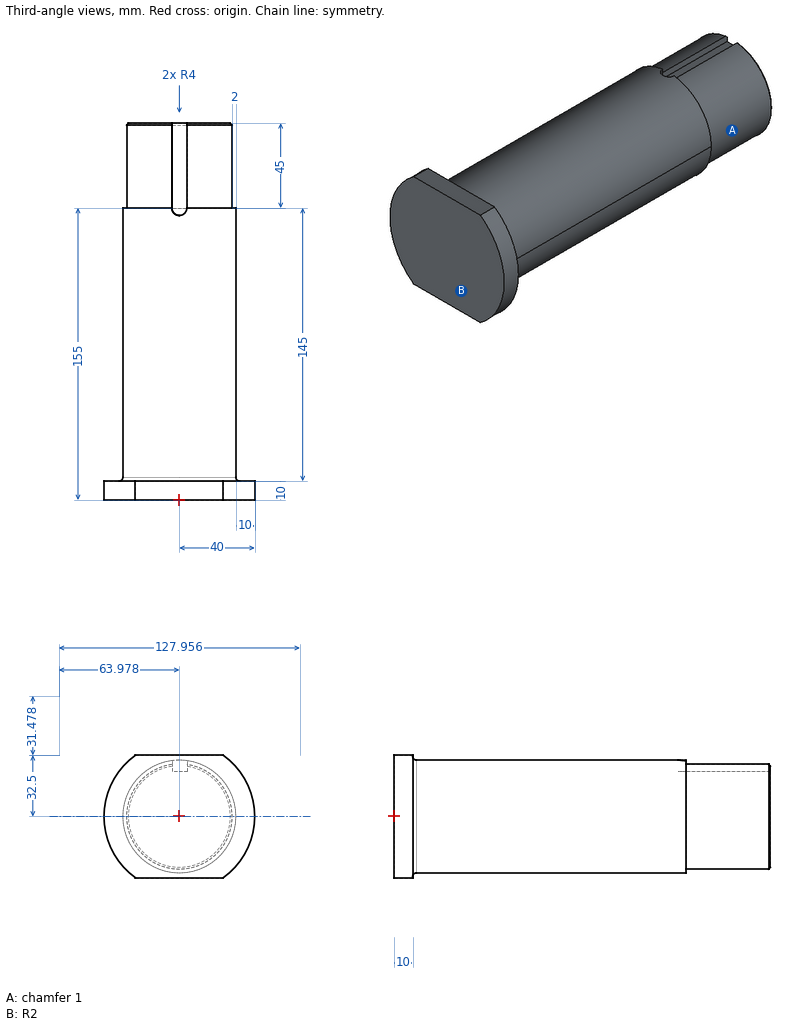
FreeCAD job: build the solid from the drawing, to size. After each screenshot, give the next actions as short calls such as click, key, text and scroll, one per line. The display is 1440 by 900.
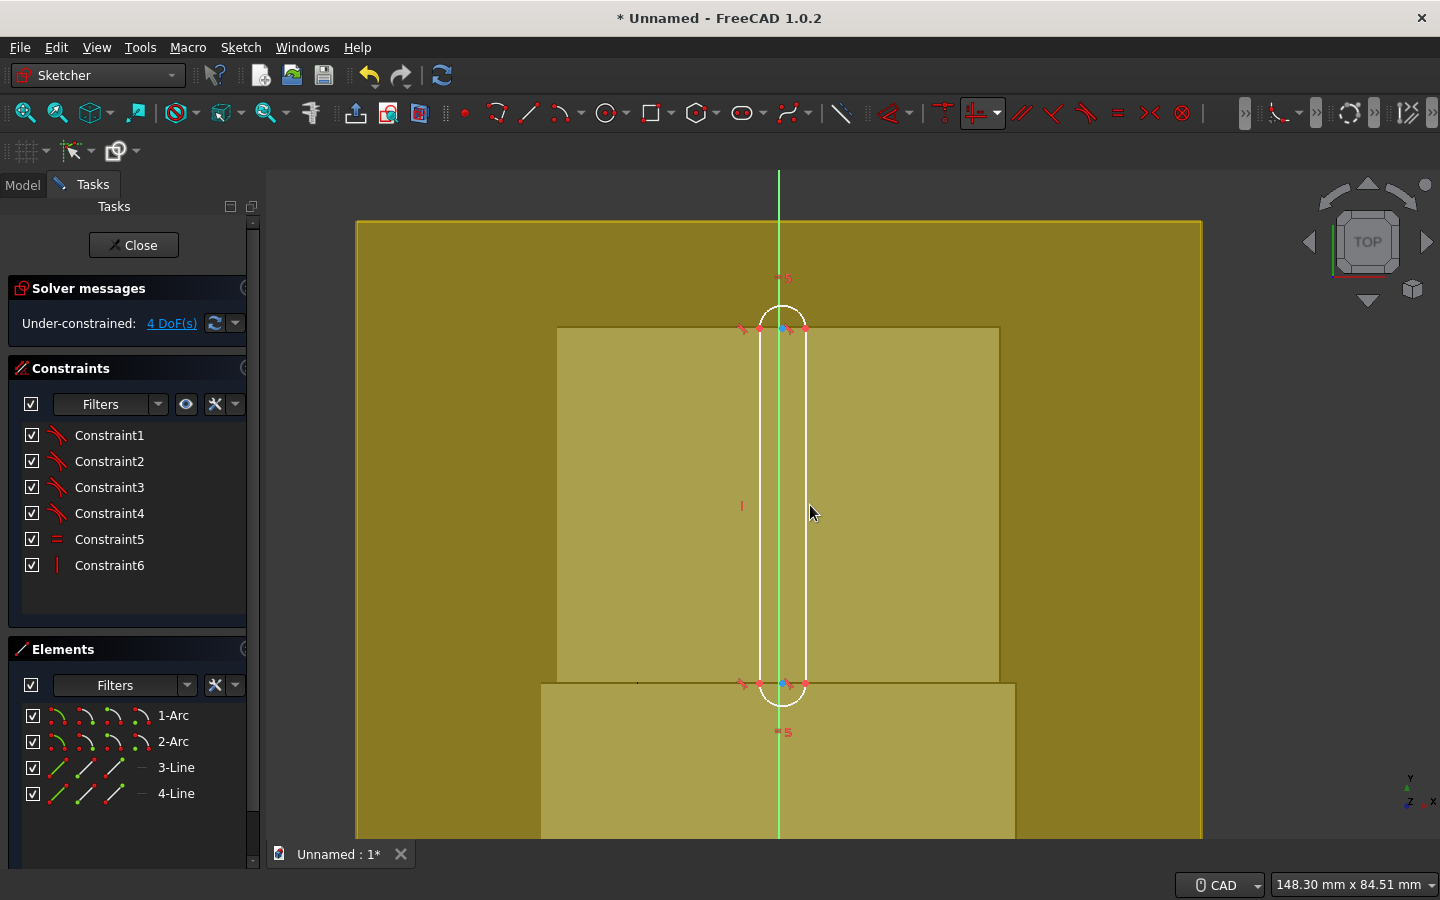
click(783, 683)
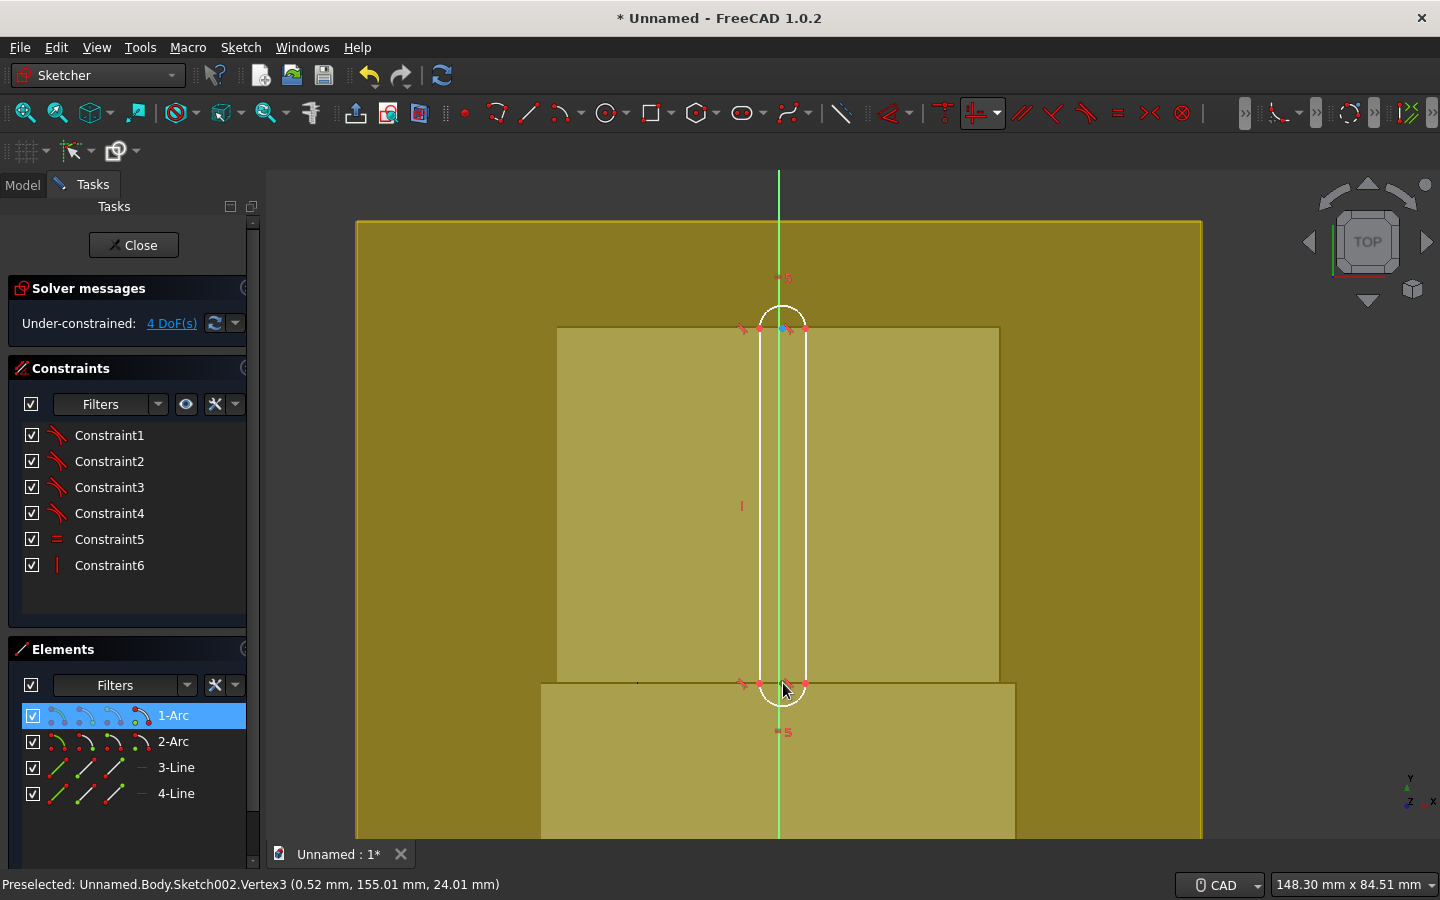
click(779, 767)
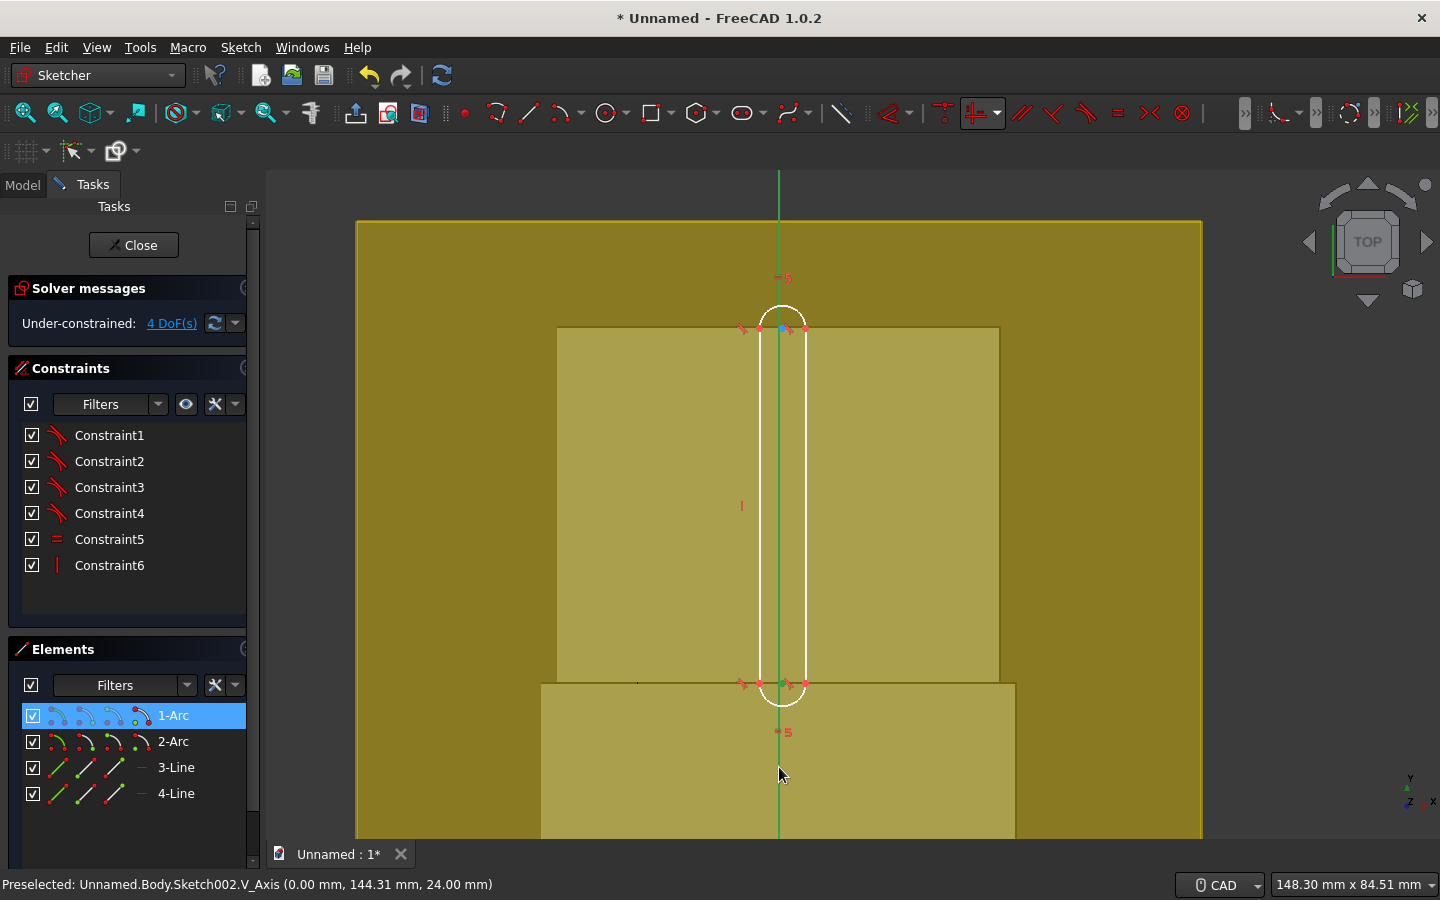
click(944, 114)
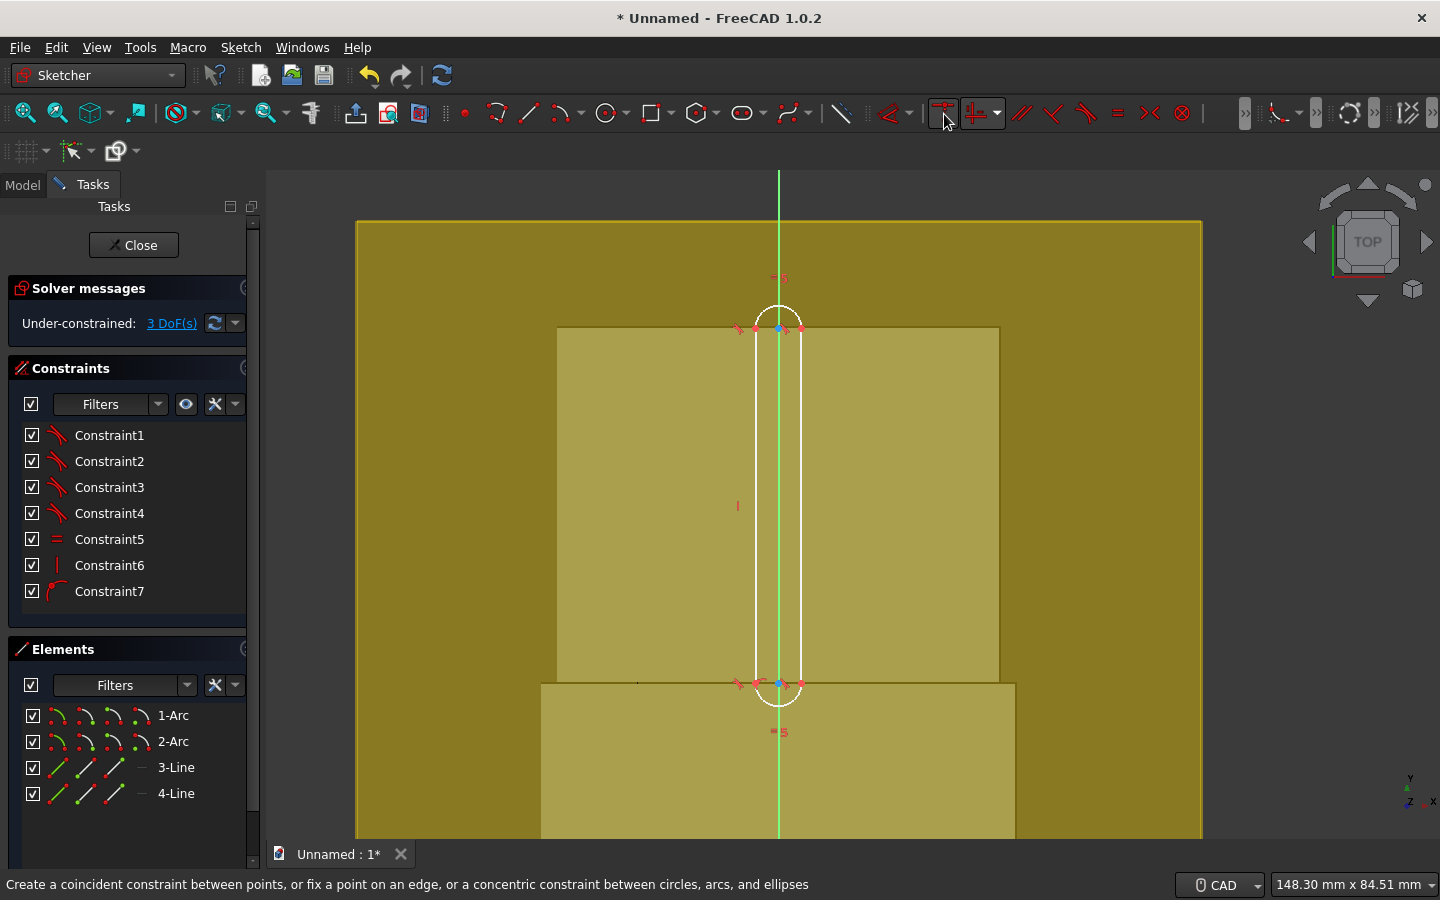
click(888, 114)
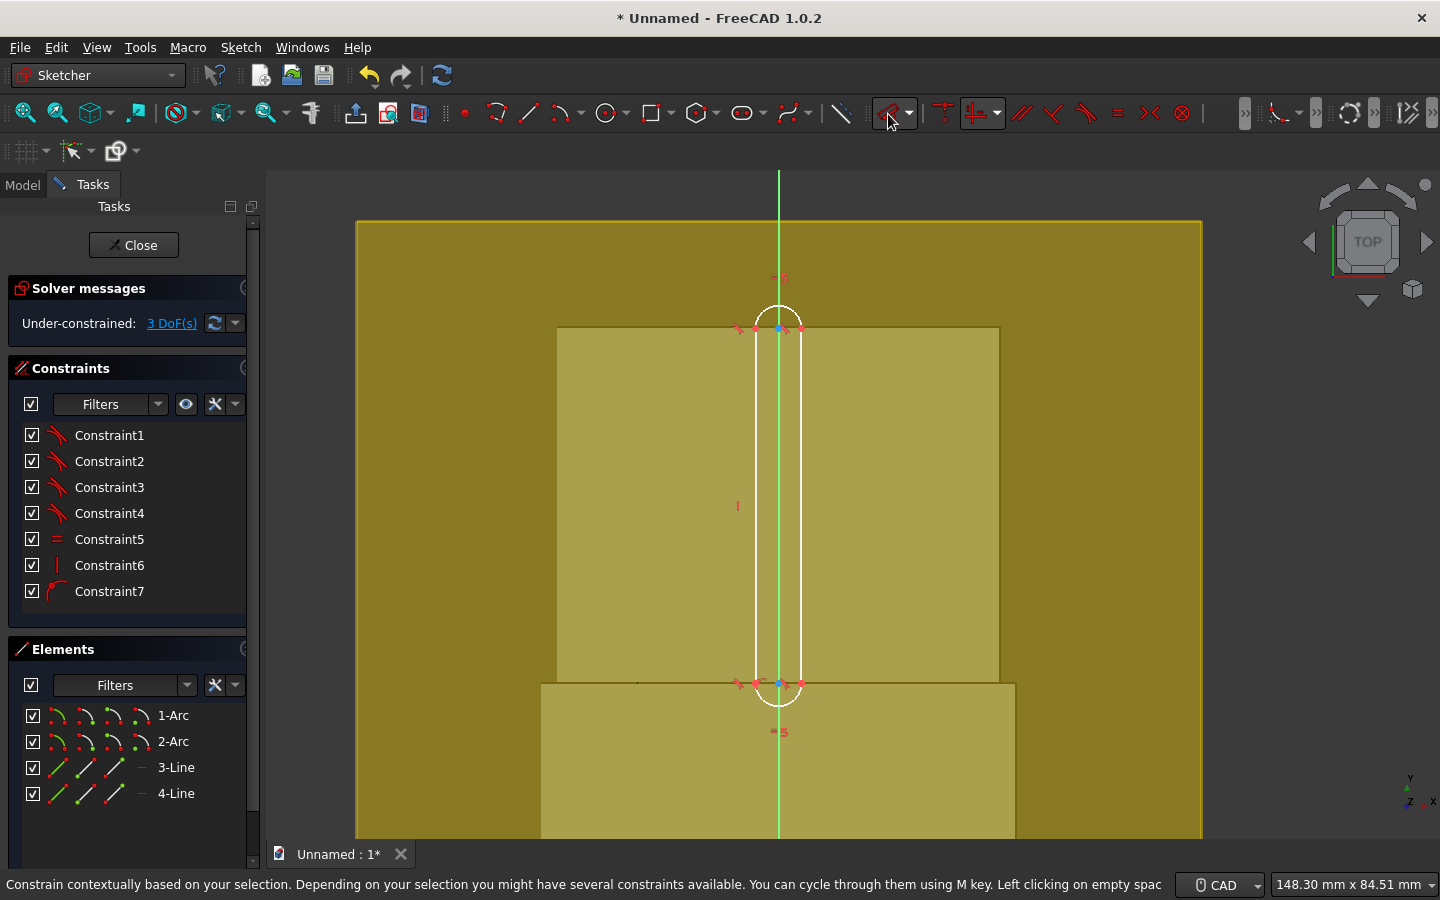
scroll(765, 702, up, 2)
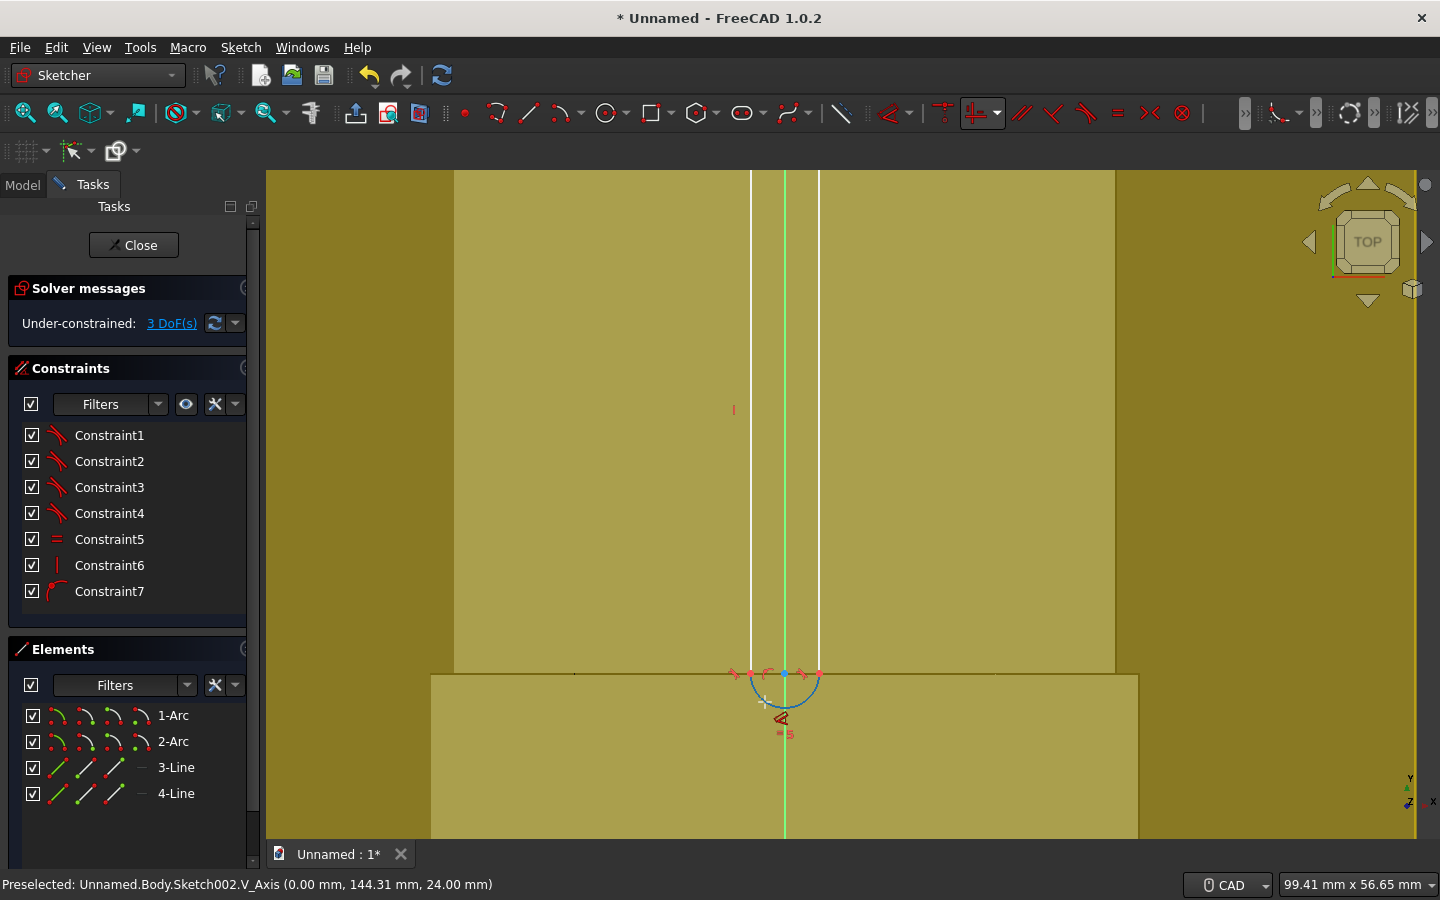
click(765, 701)
click(746, 727)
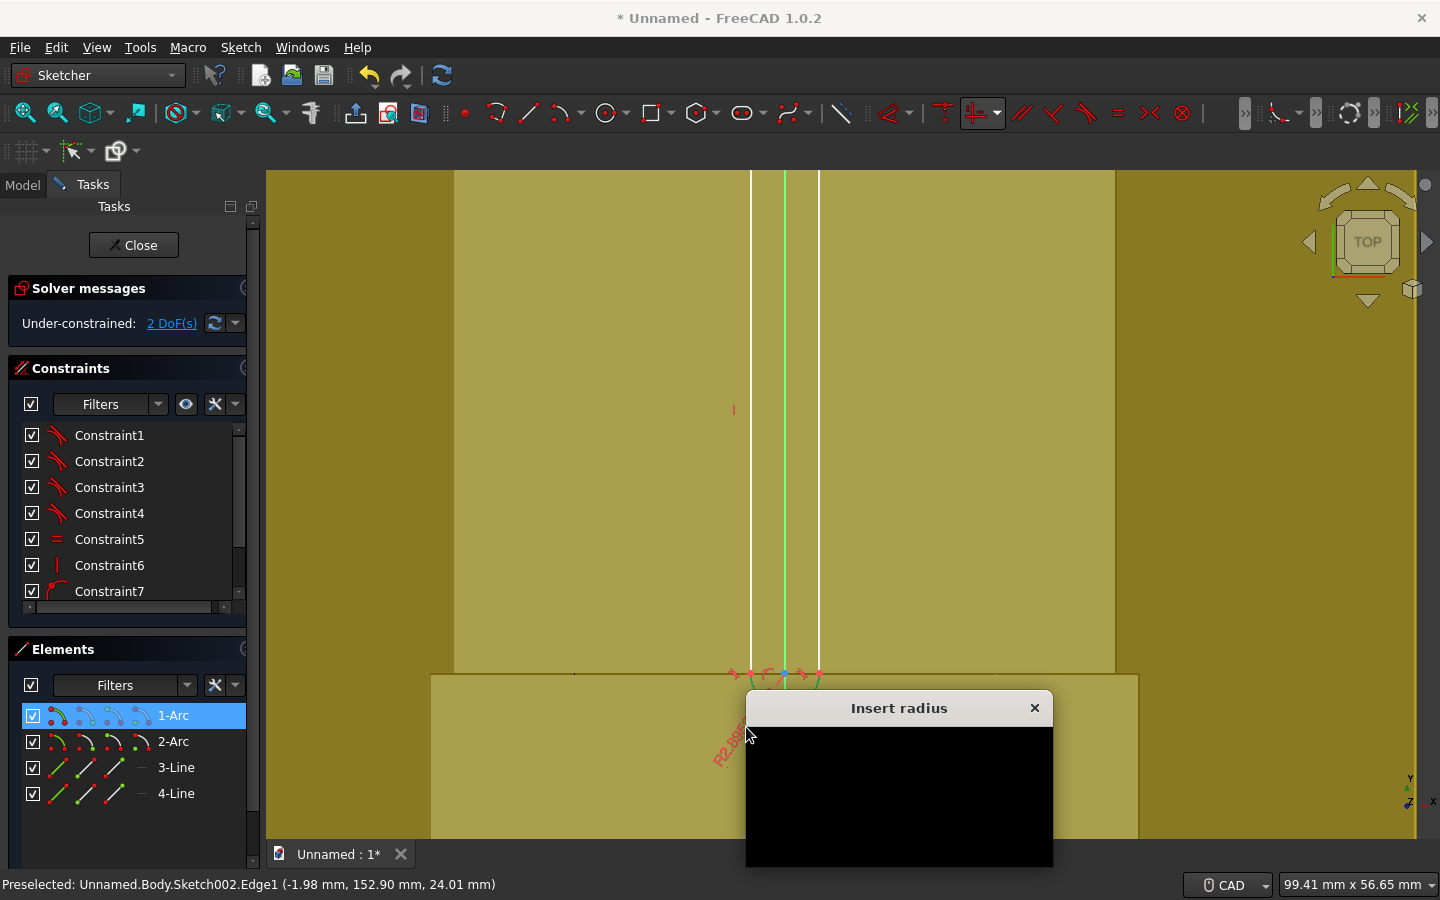
text(4)
key(Return)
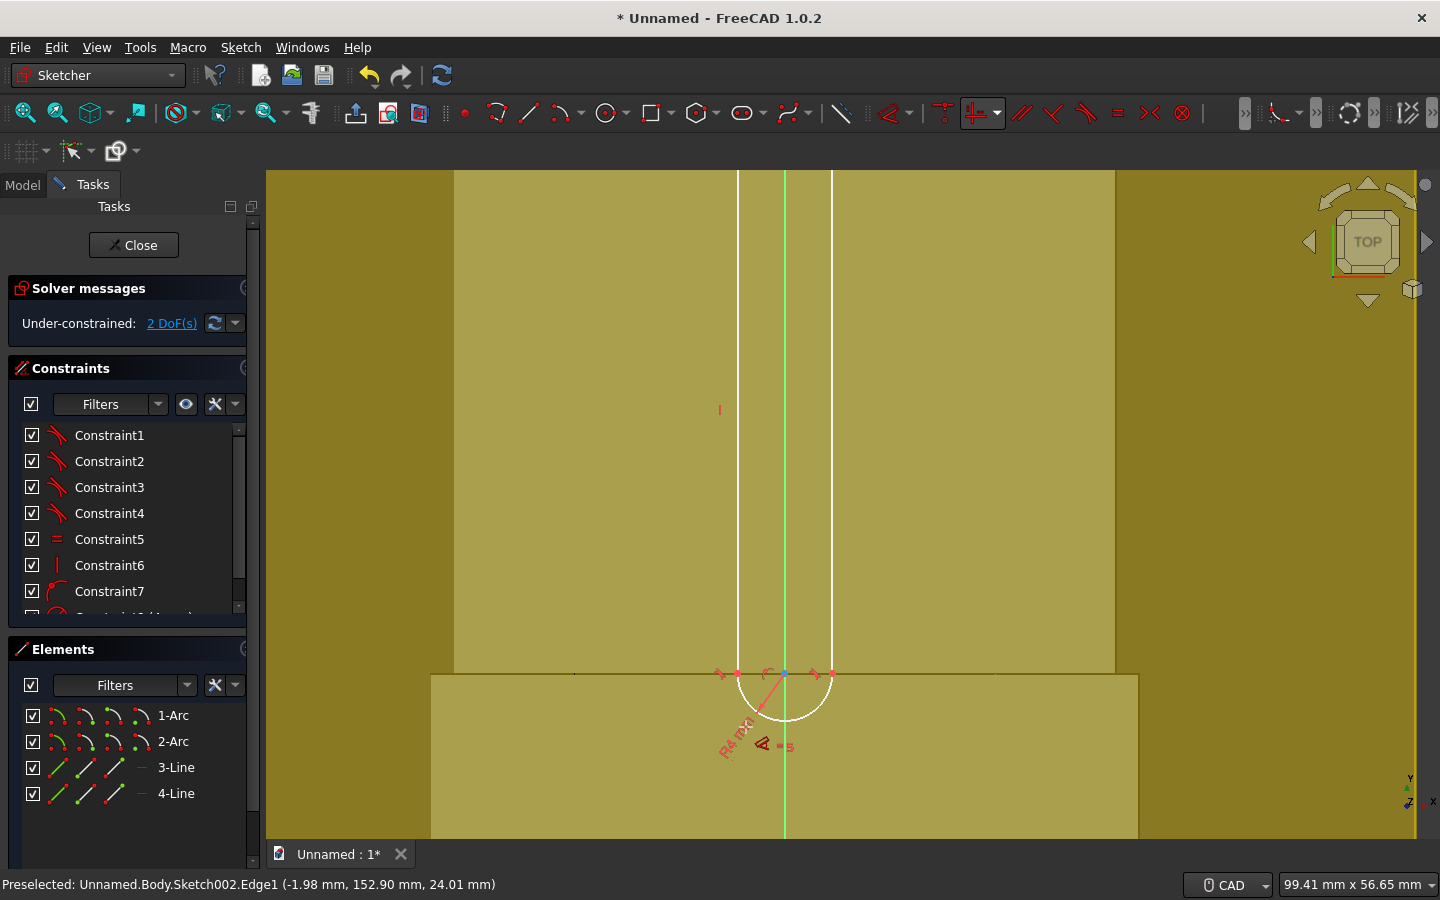
click(738, 515)
click(704, 436)